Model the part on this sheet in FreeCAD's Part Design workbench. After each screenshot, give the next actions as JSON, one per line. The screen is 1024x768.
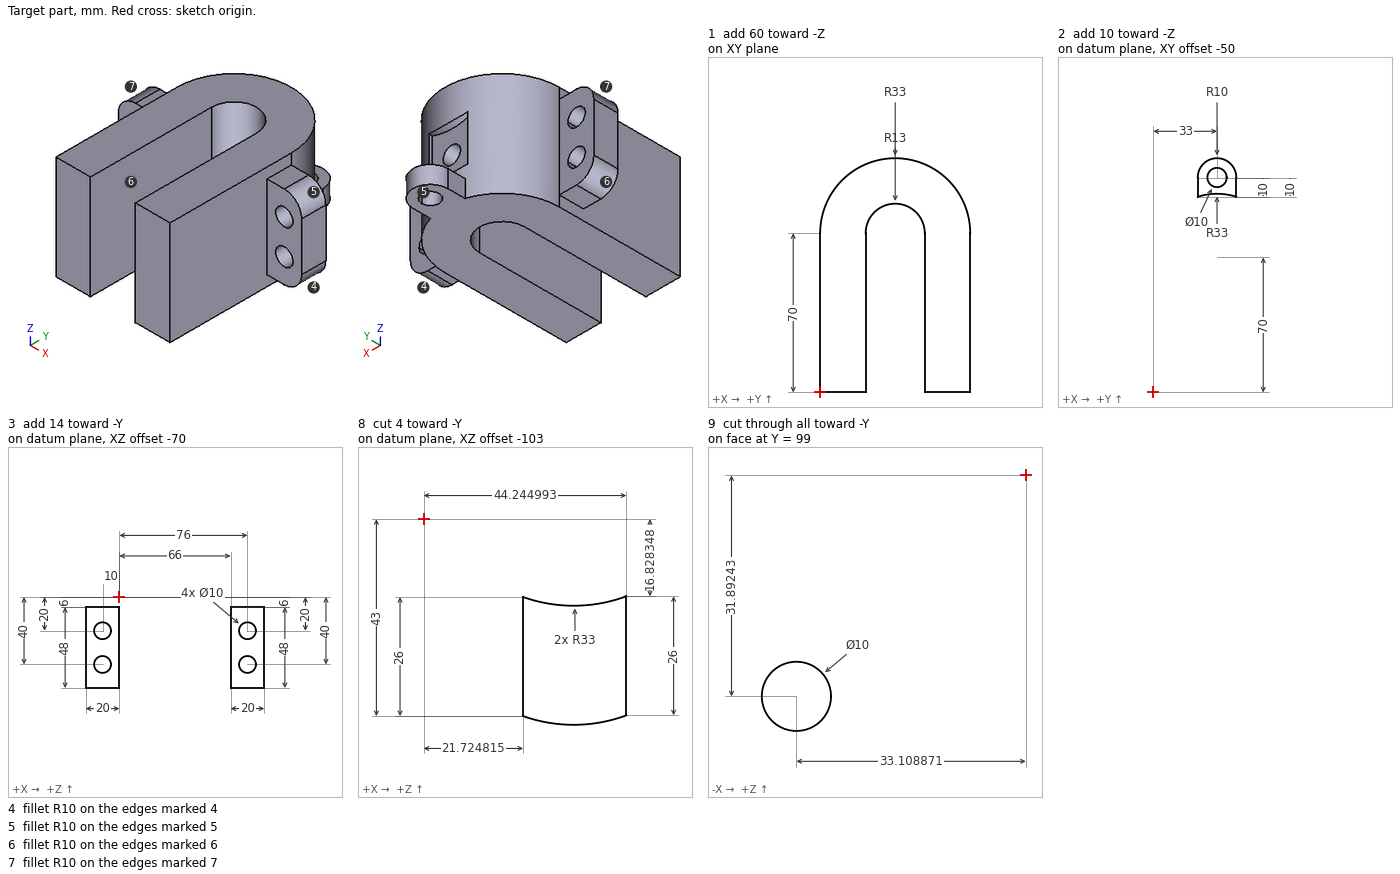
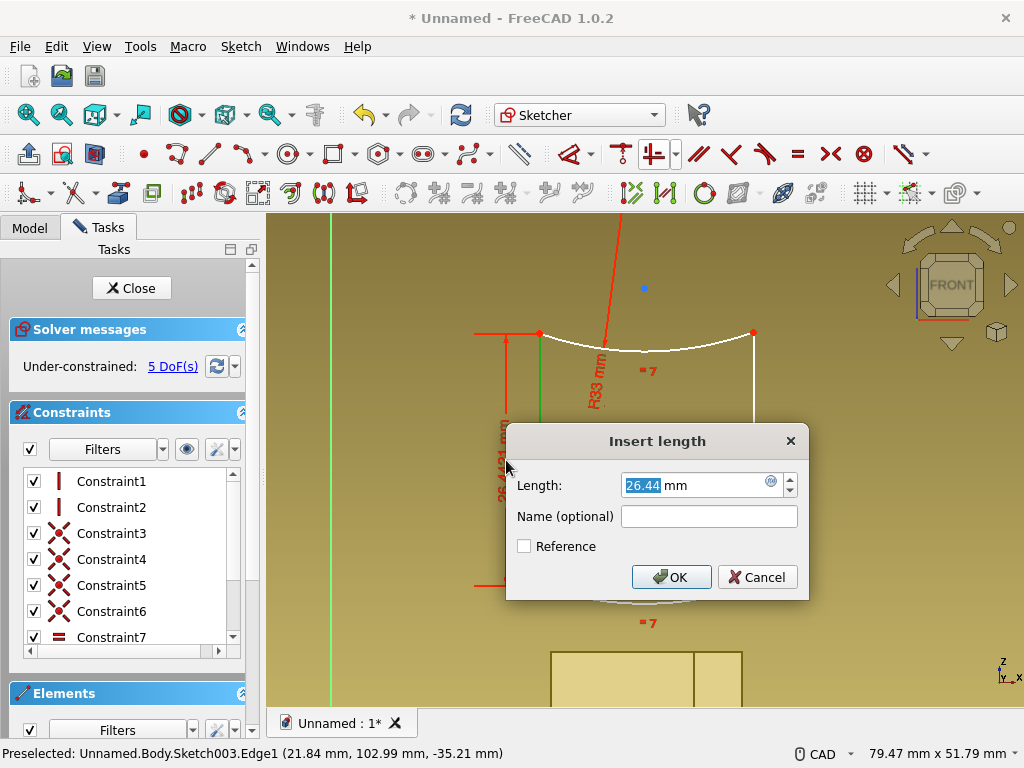
{"action": "type", "text": "26"}
{"action": "key", "text": "Return"}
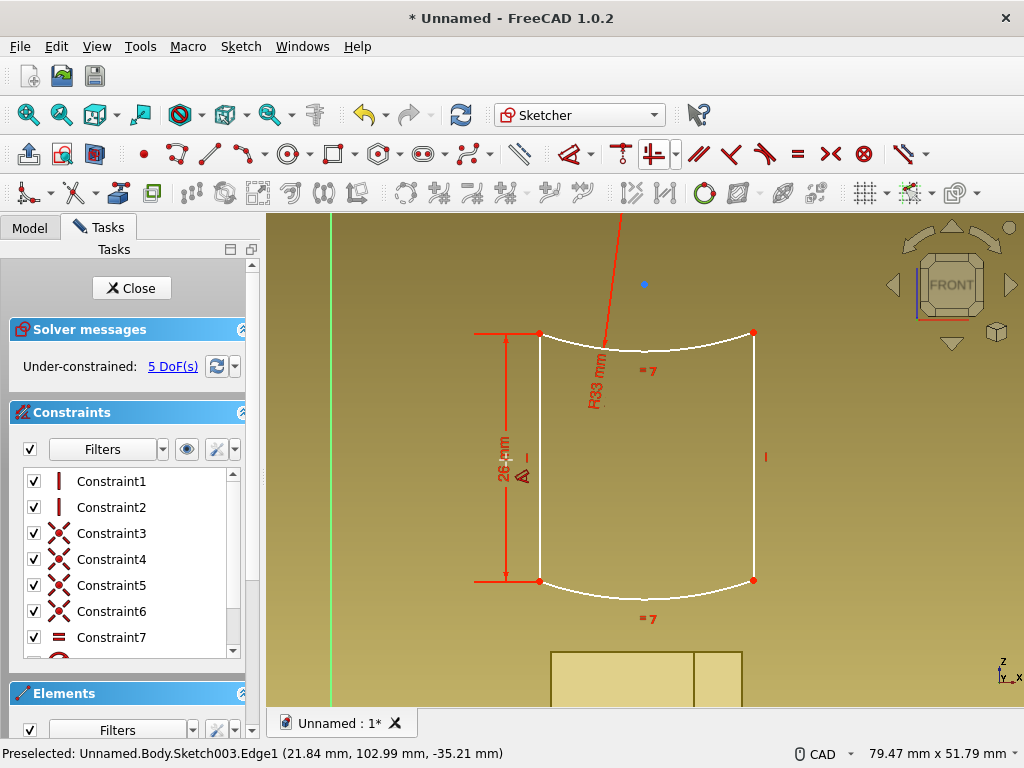
{"action": "left_click", "coordinate": [754, 406]}
{"action": "left_click", "coordinate": [788, 456]}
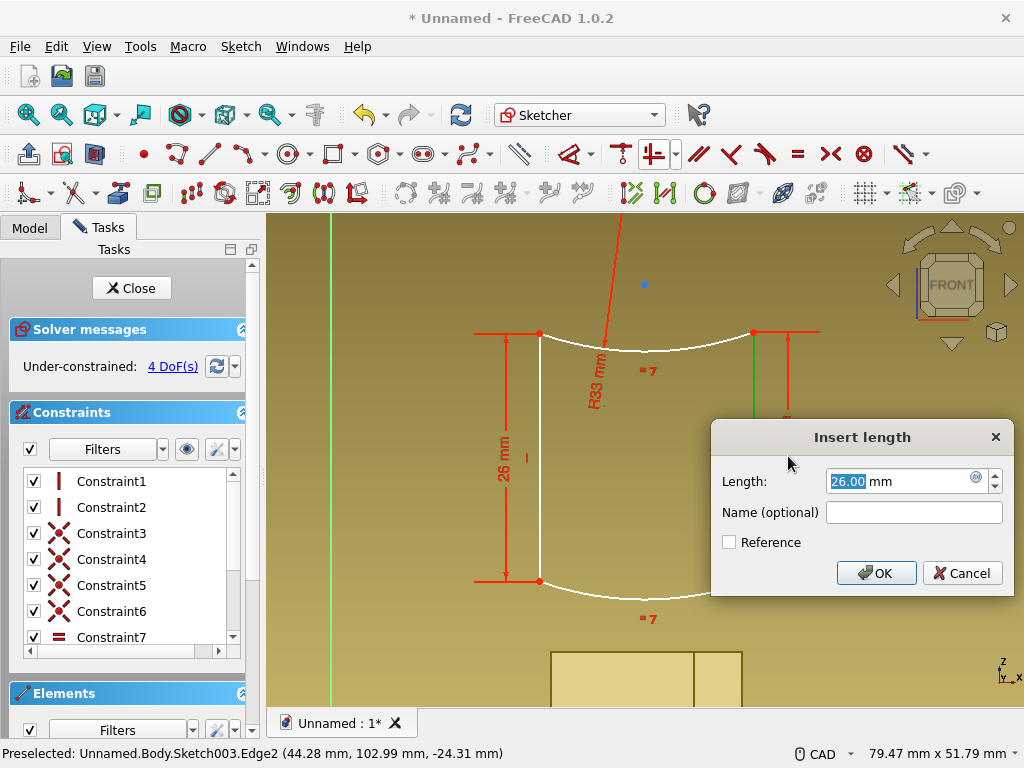
{"action": "type", "text": "26"}
{"action": "key", "text": "Return"}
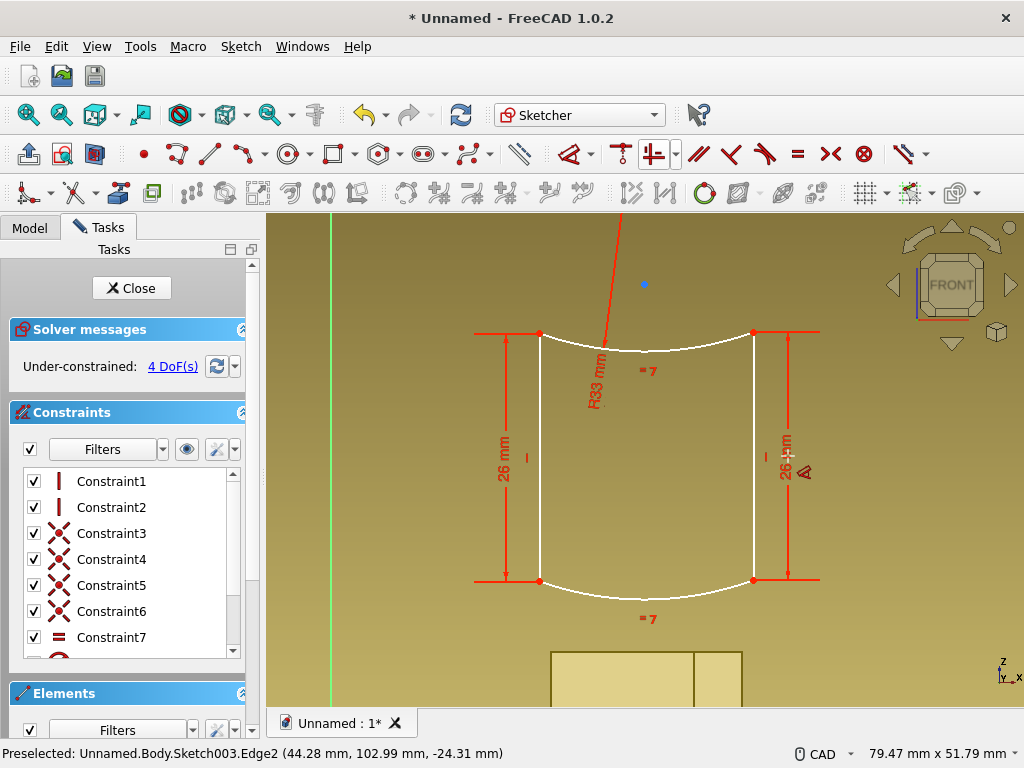
{"action": "left_click", "coordinate": [540, 582]}
{"action": "left_click", "coordinate": [297, 411]}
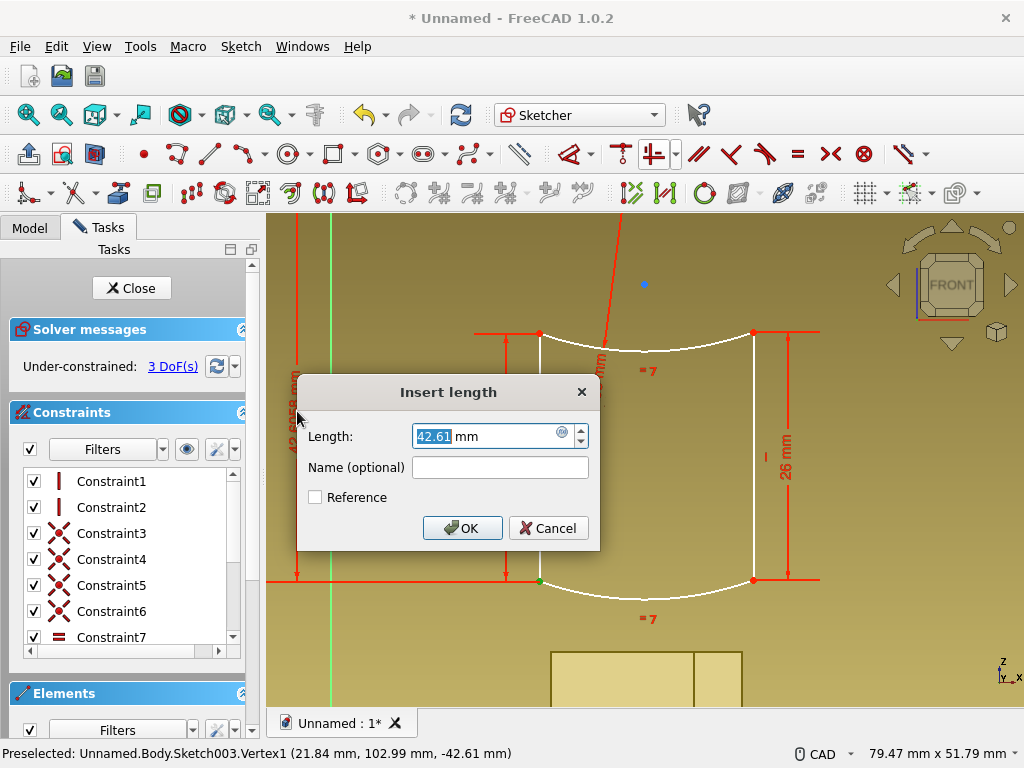
{"action": "type", "text": "43"}
{"action": "key", "text": "Return"}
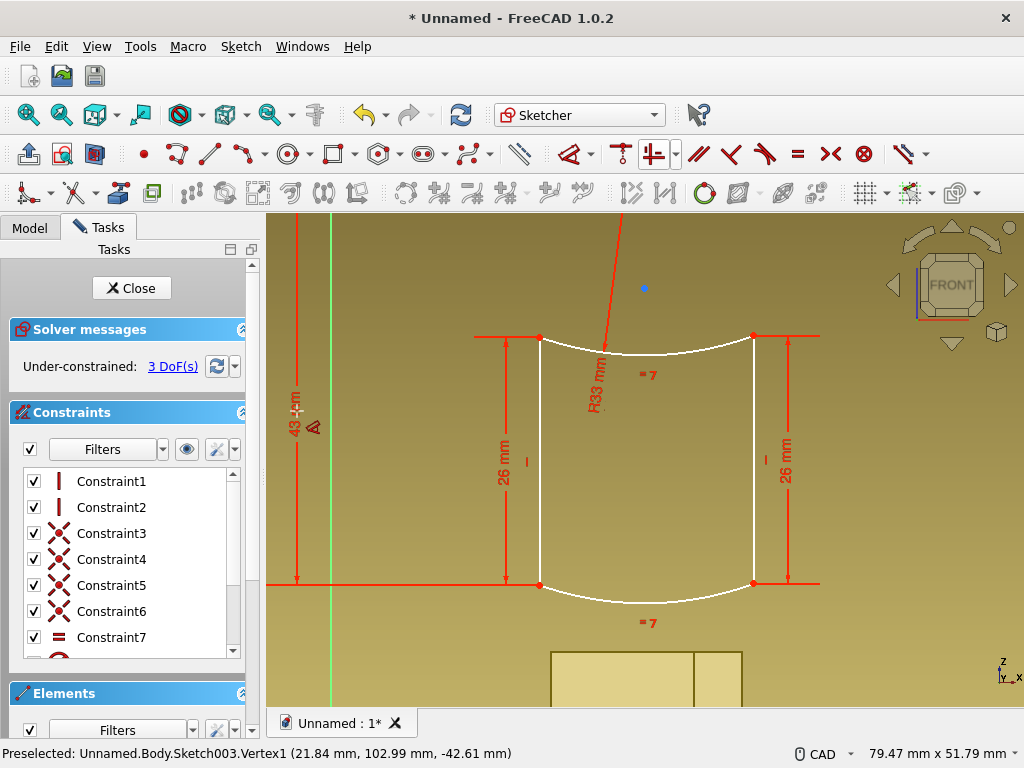
{"action": "left_click", "coordinate": [540, 585]}
{"action": "left_click", "coordinate": [436, 619]}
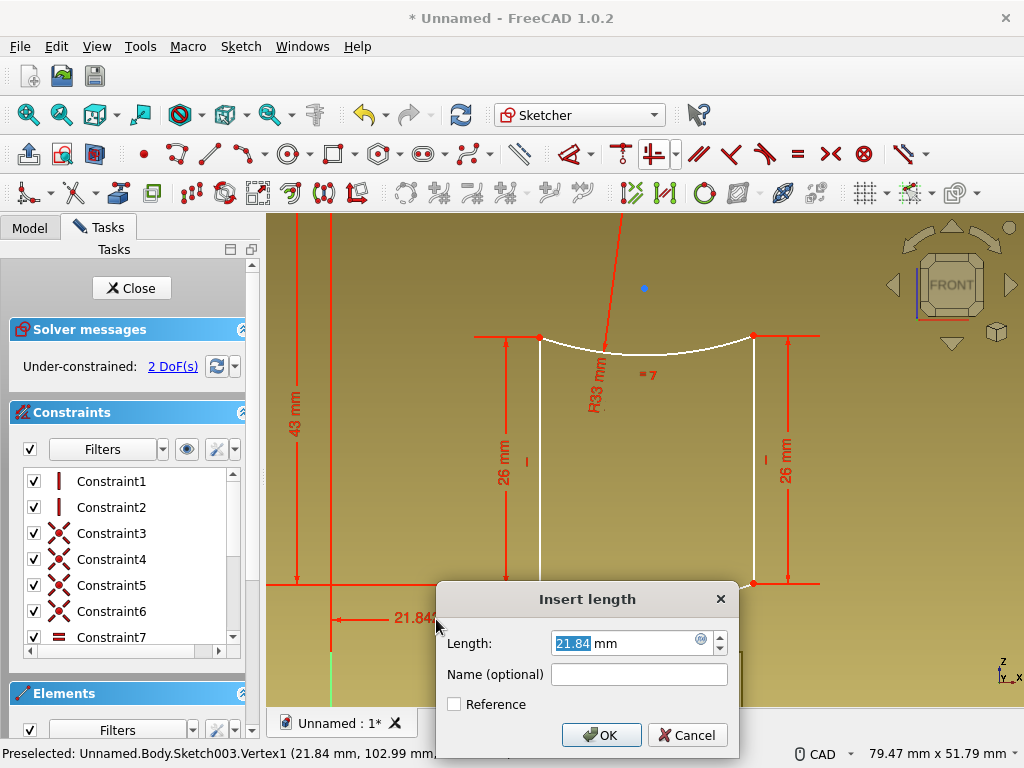
{"action": "type", "text": "21.724815"}
{"action": "key", "text": "Return"}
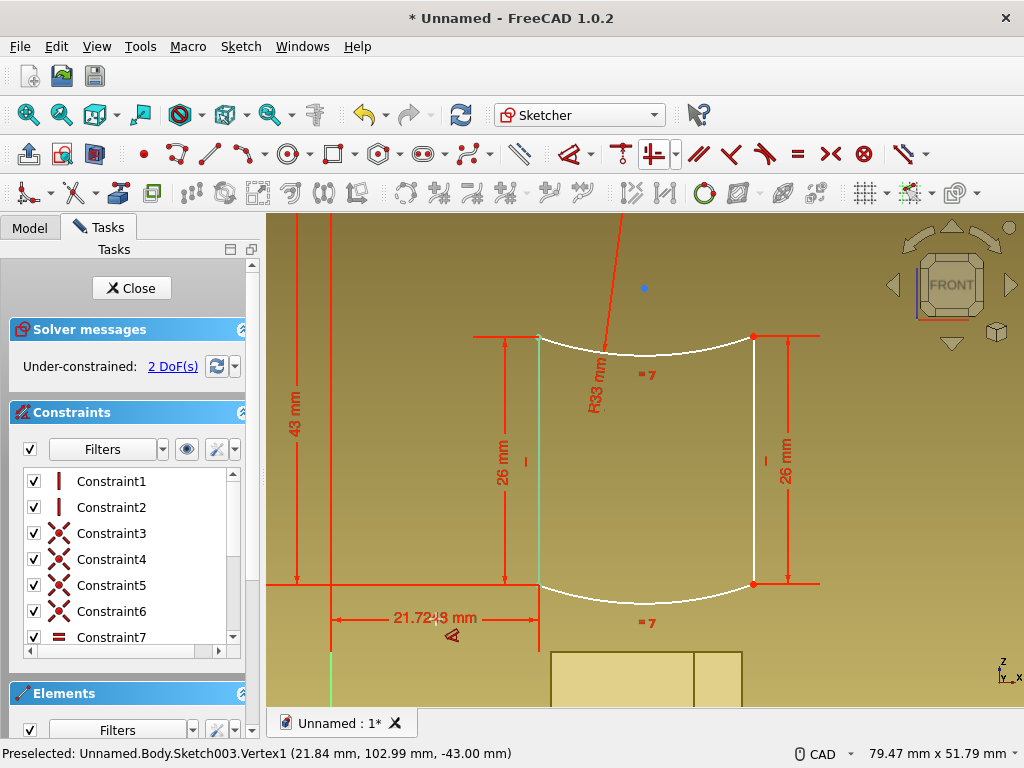
{"action": "left_click", "coordinate": [754, 336]}
{"action": "left_click", "coordinate": [445, 370]}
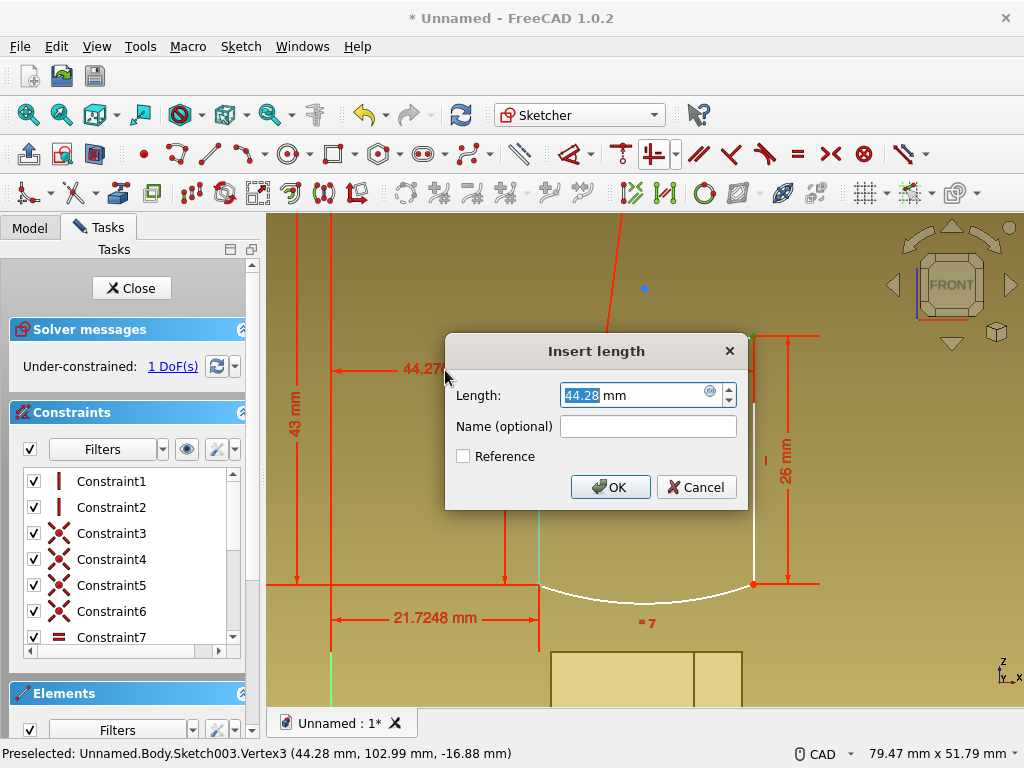
{"action": "type", "text": "44.244993"}
{"action": "key", "text": "Return"}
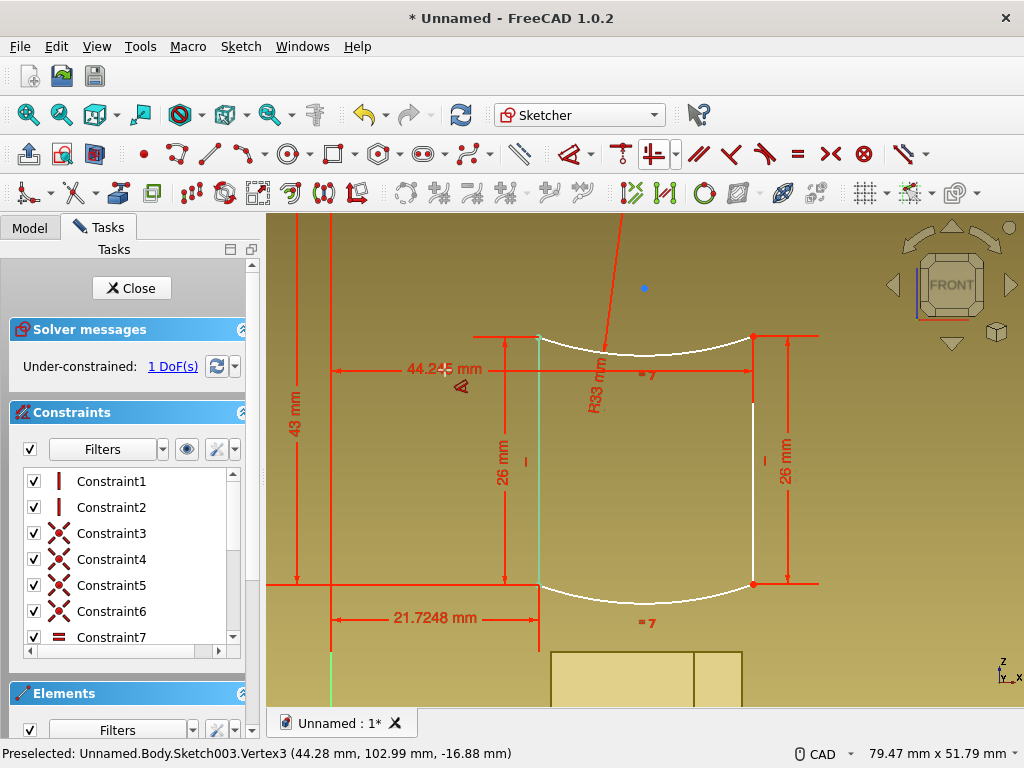
{"action": "left_click", "coordinate": [753, 336]}
{"action": "left_click", "coordinate": [297, 289]}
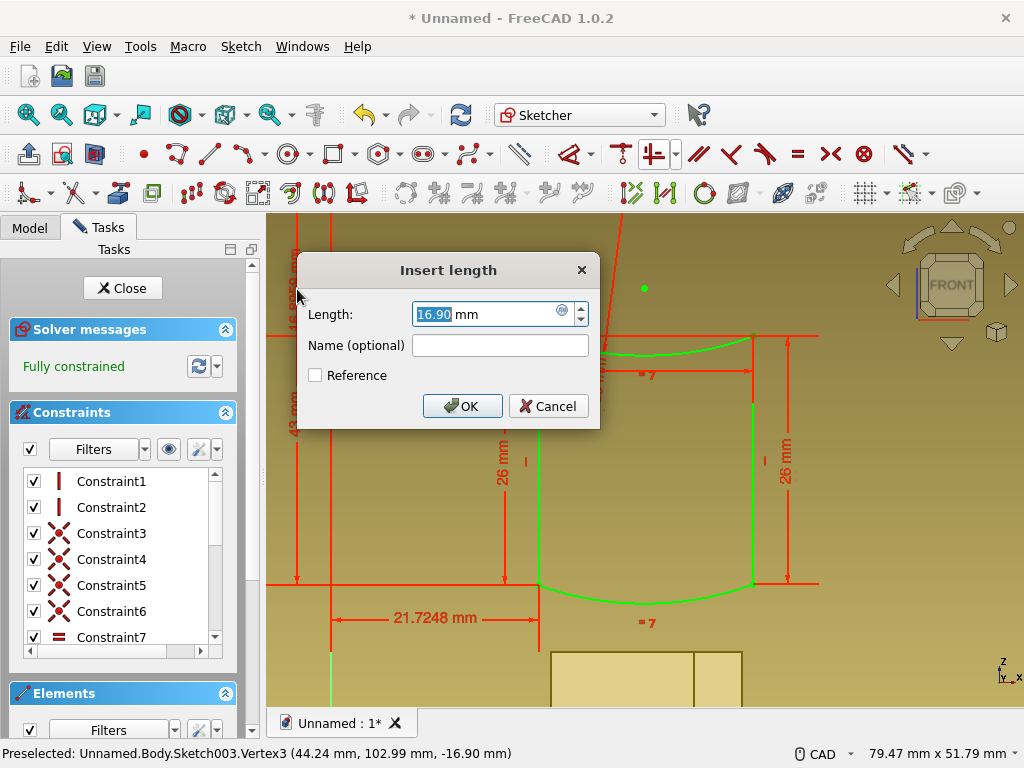
{"action": "type", "text": "16.828348"}
{"action": "key", "text": "Return"}
{"action": "key", "text": "Escape"}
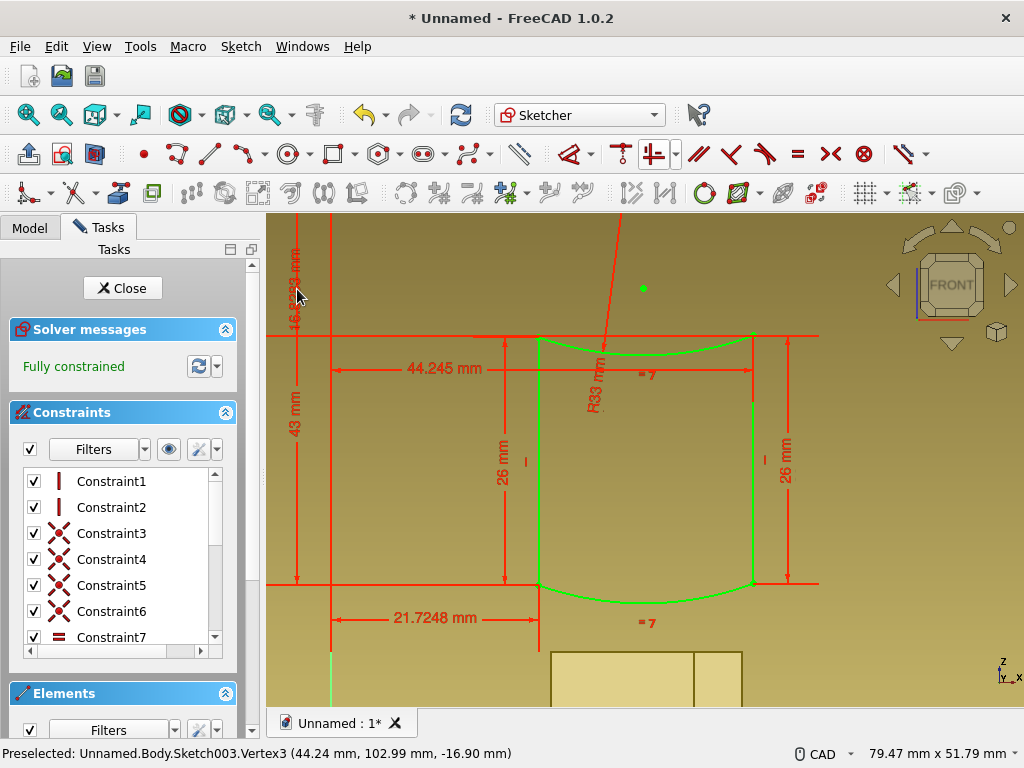
{"action": "left_click", "coordinate": [123, 288]}